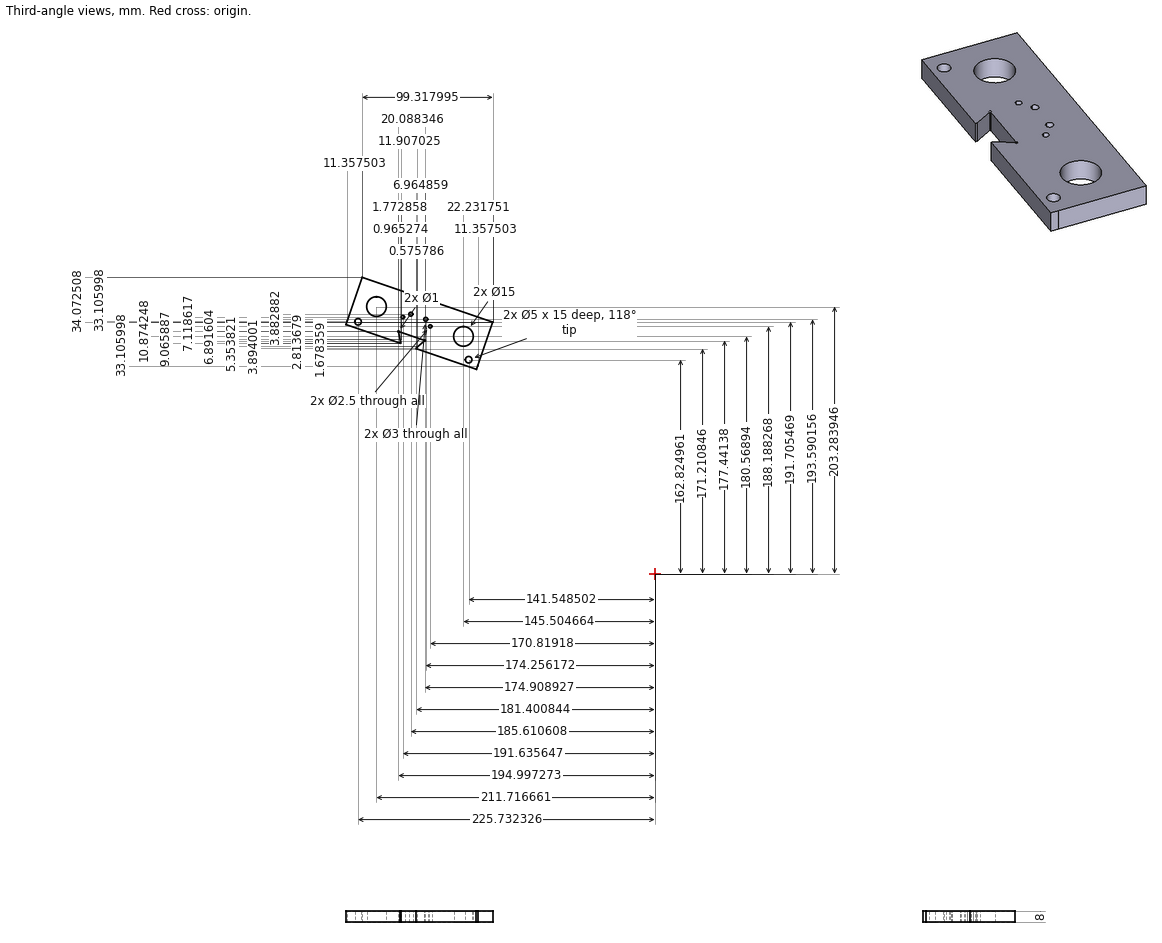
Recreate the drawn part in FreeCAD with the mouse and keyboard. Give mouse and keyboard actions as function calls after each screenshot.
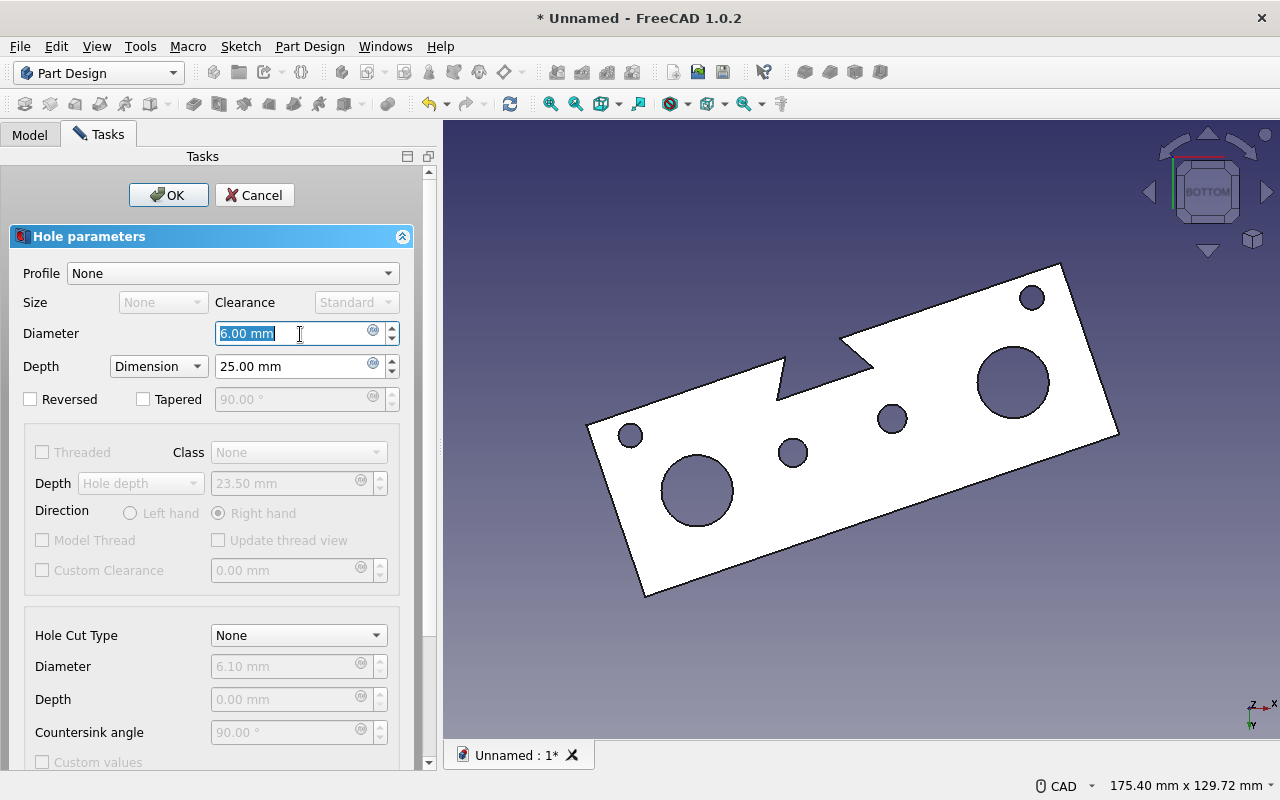
text(2.5)
key(Tab)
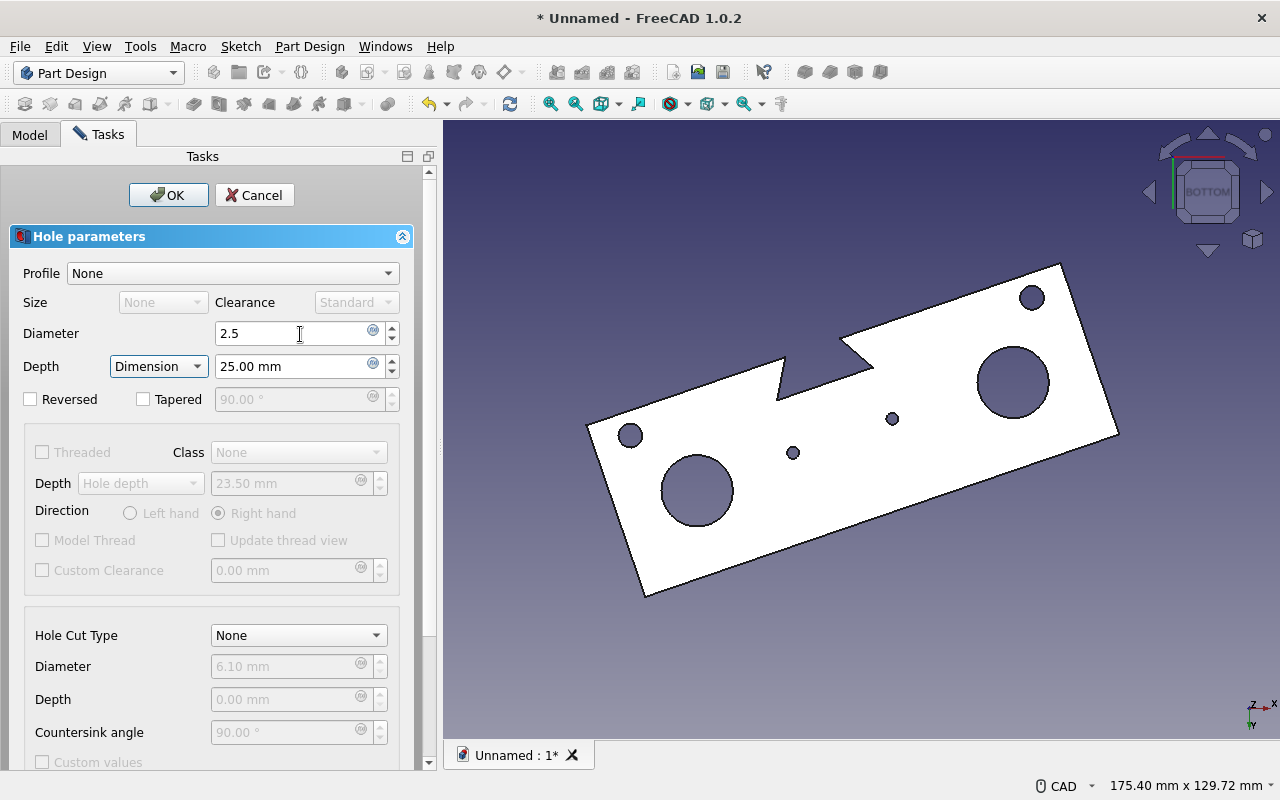
click(160, 366)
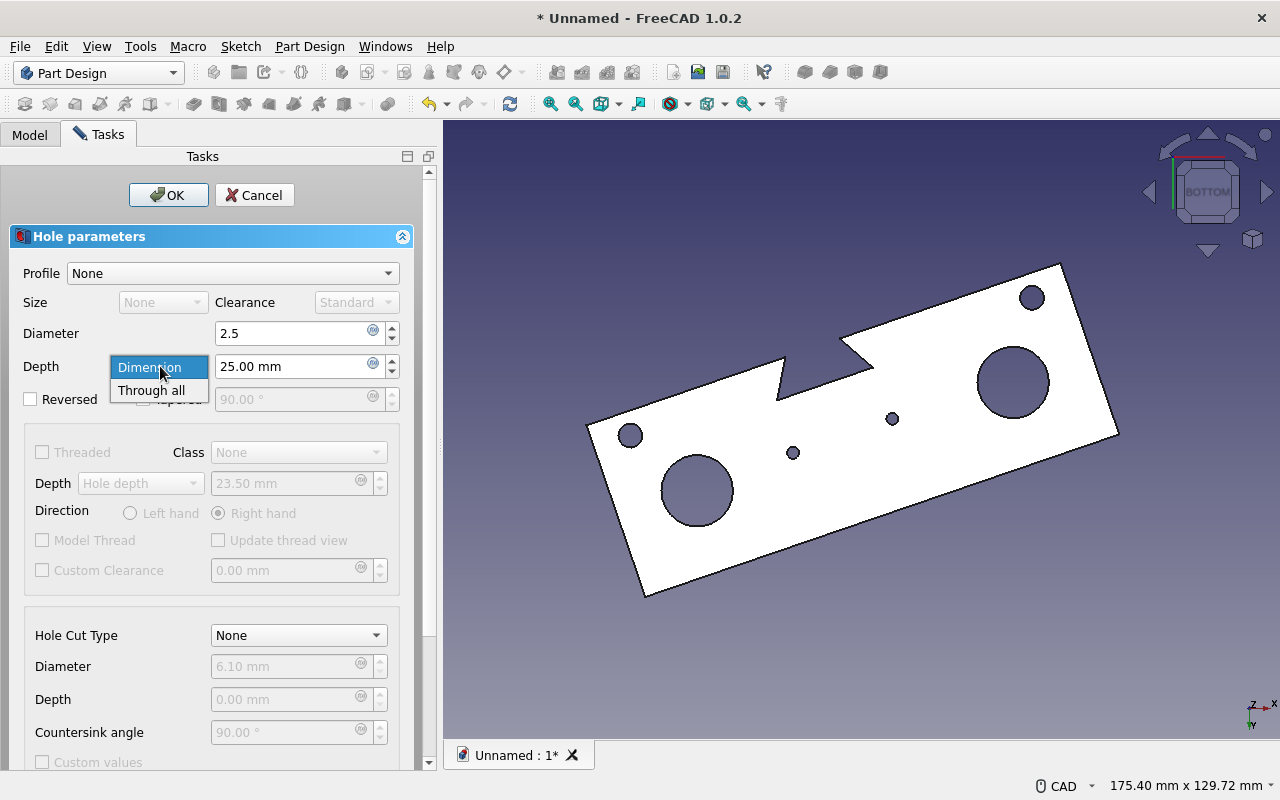
click(158, 390)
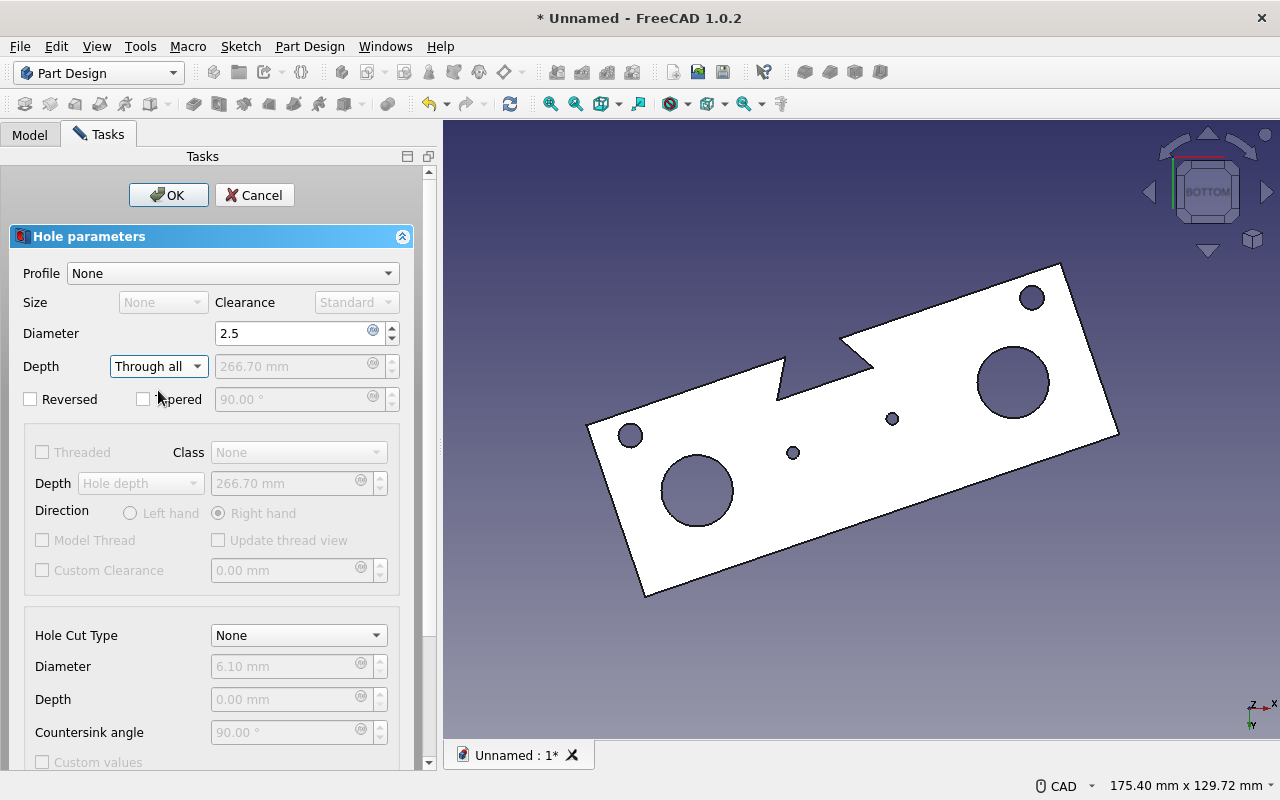
click(169, 195)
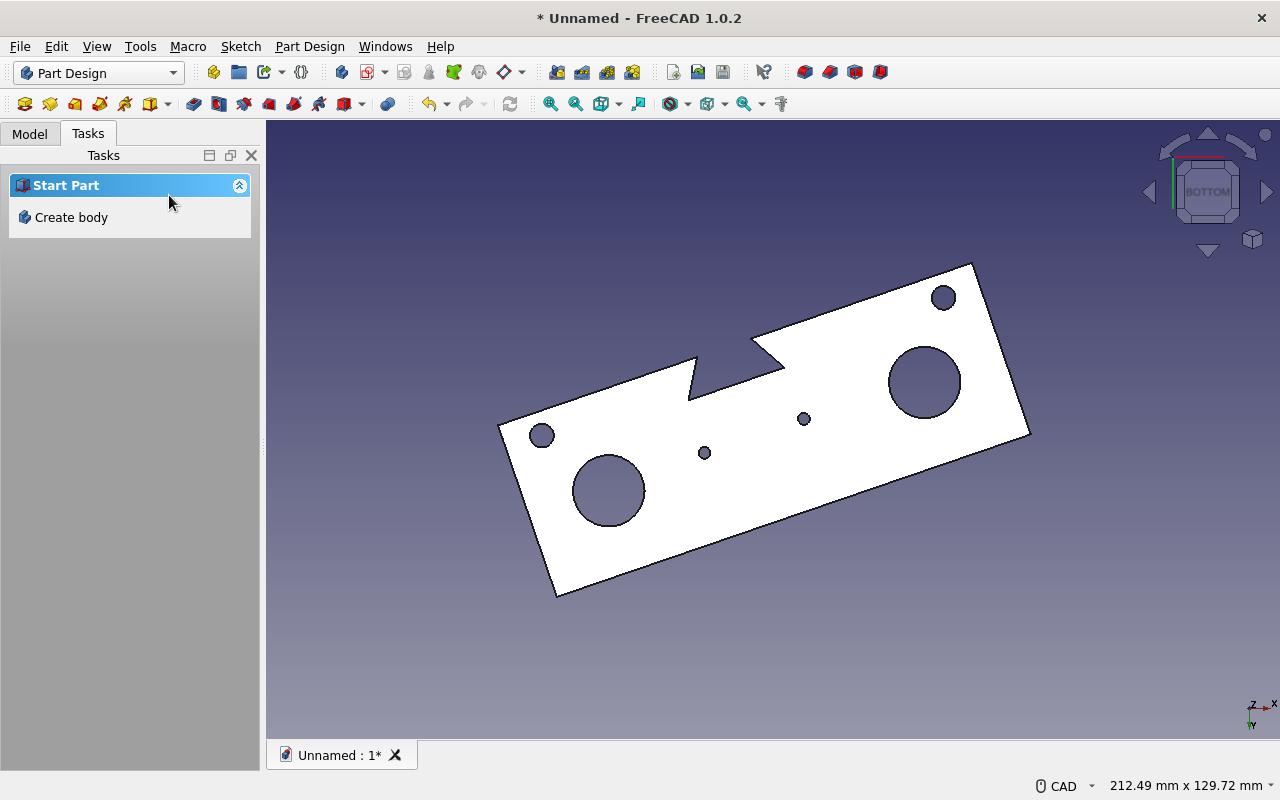
click(840, 381)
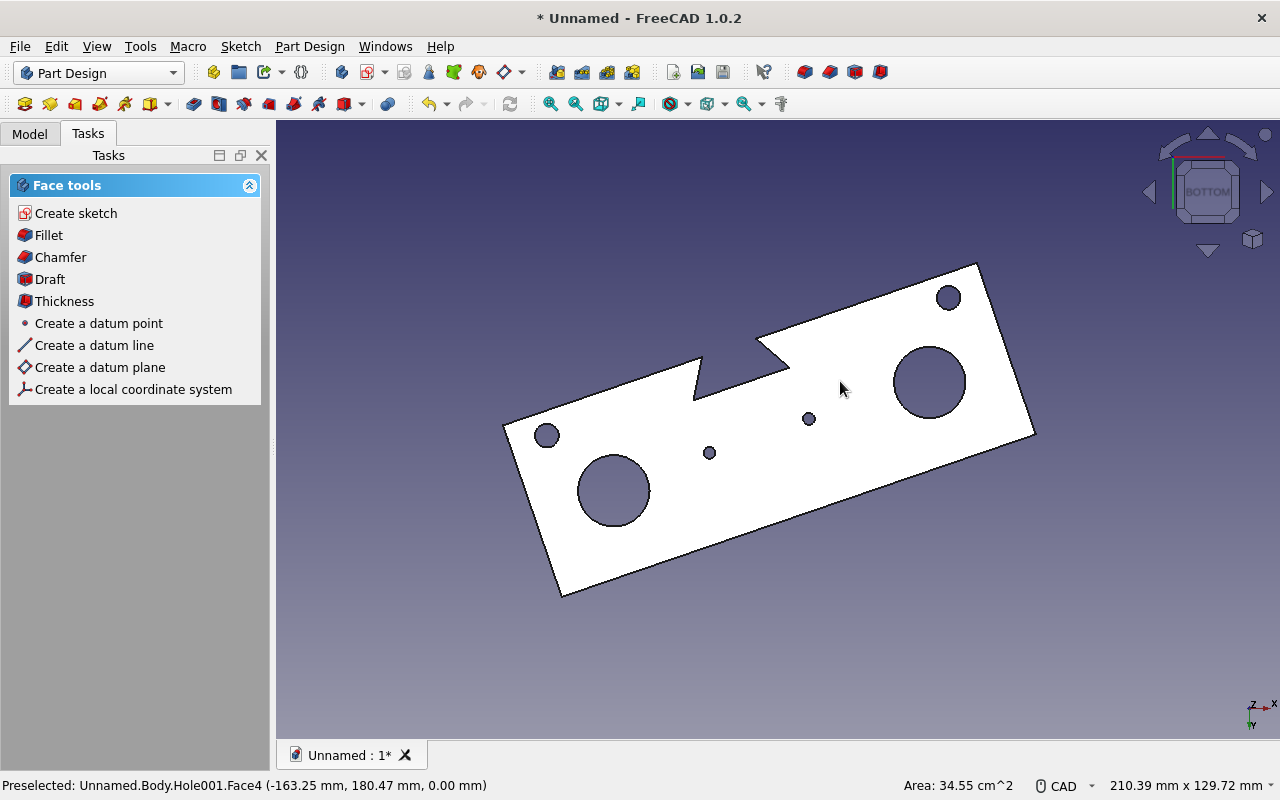
click(366, 72)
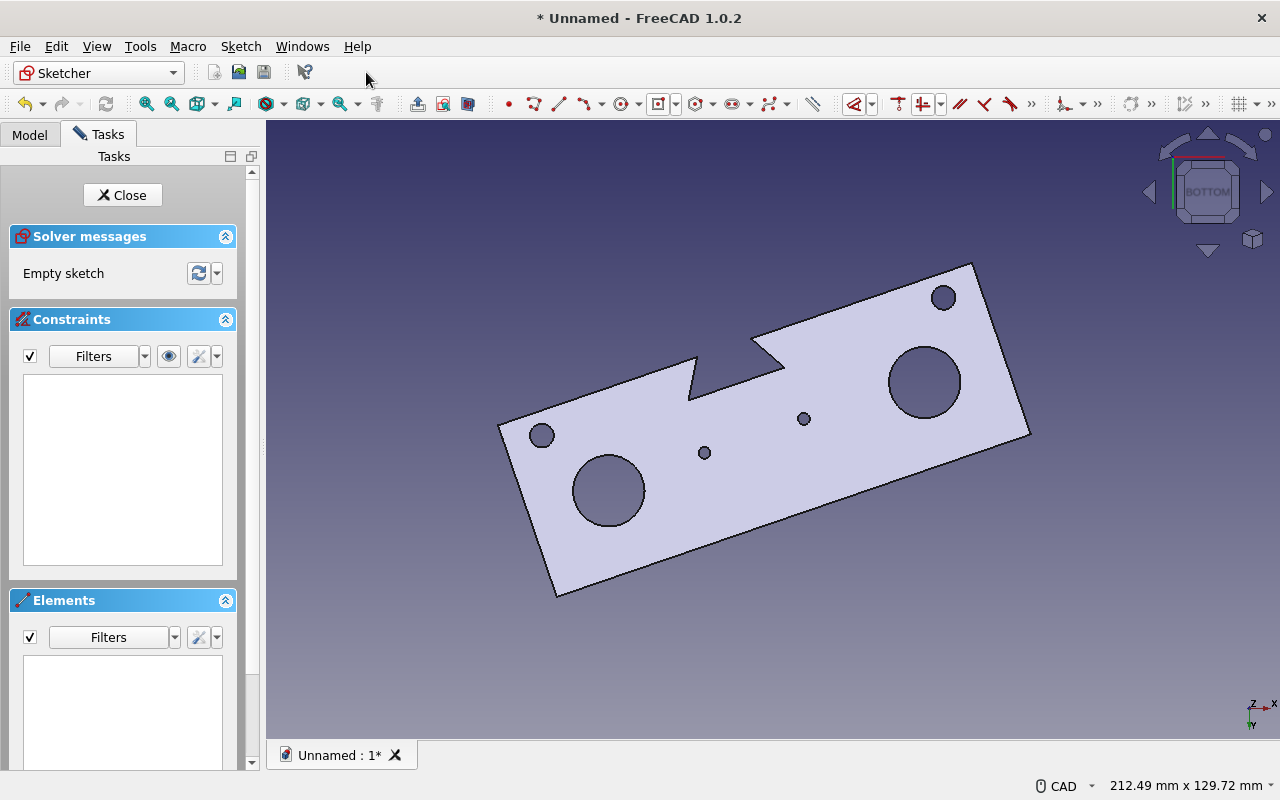
scroll(767, 457, up, 11)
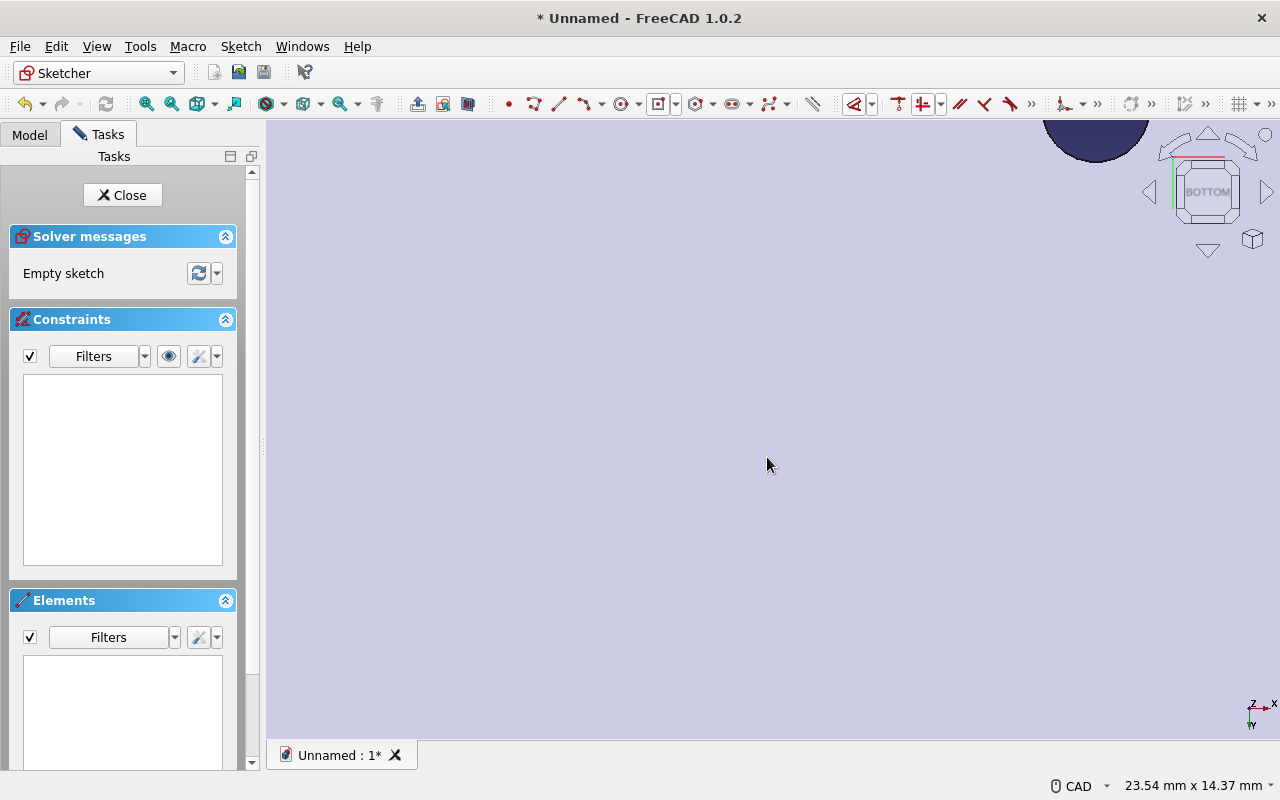
click(620, 104)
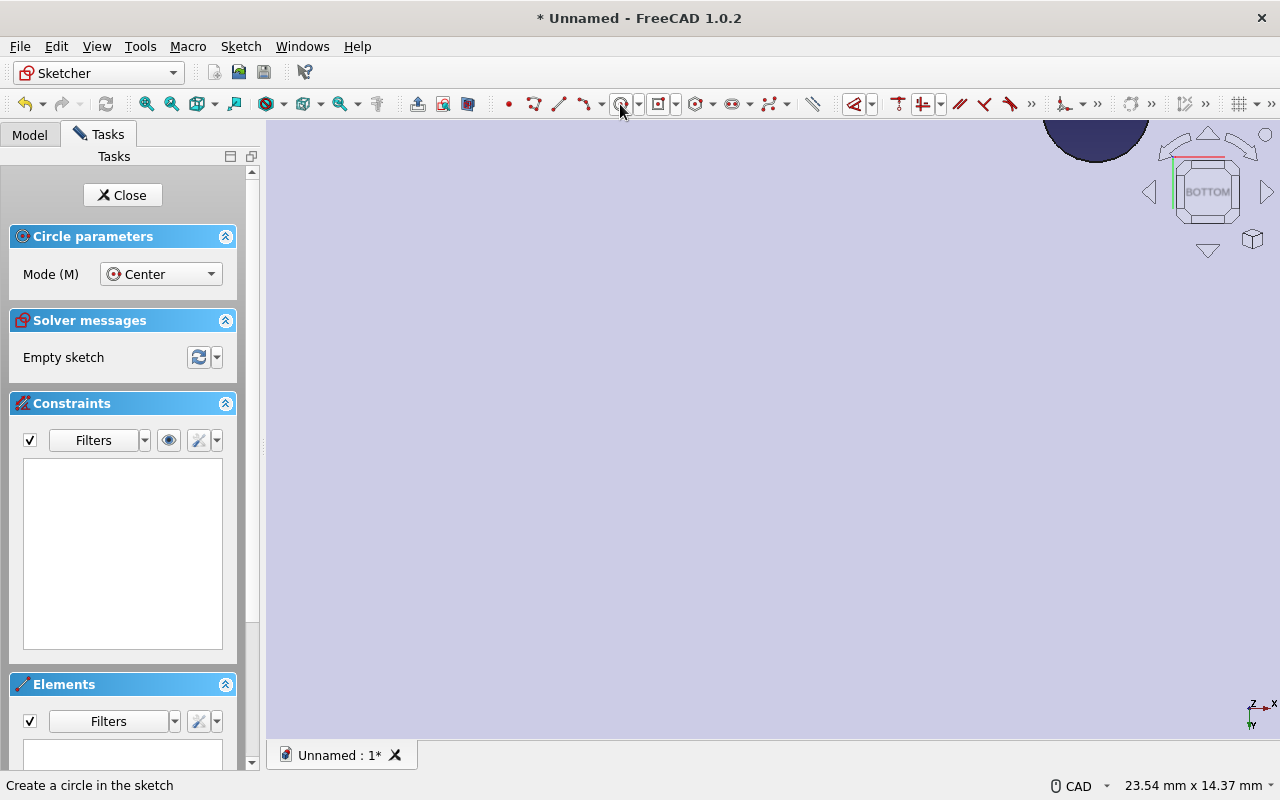
click(948, 341)
click(994, 295)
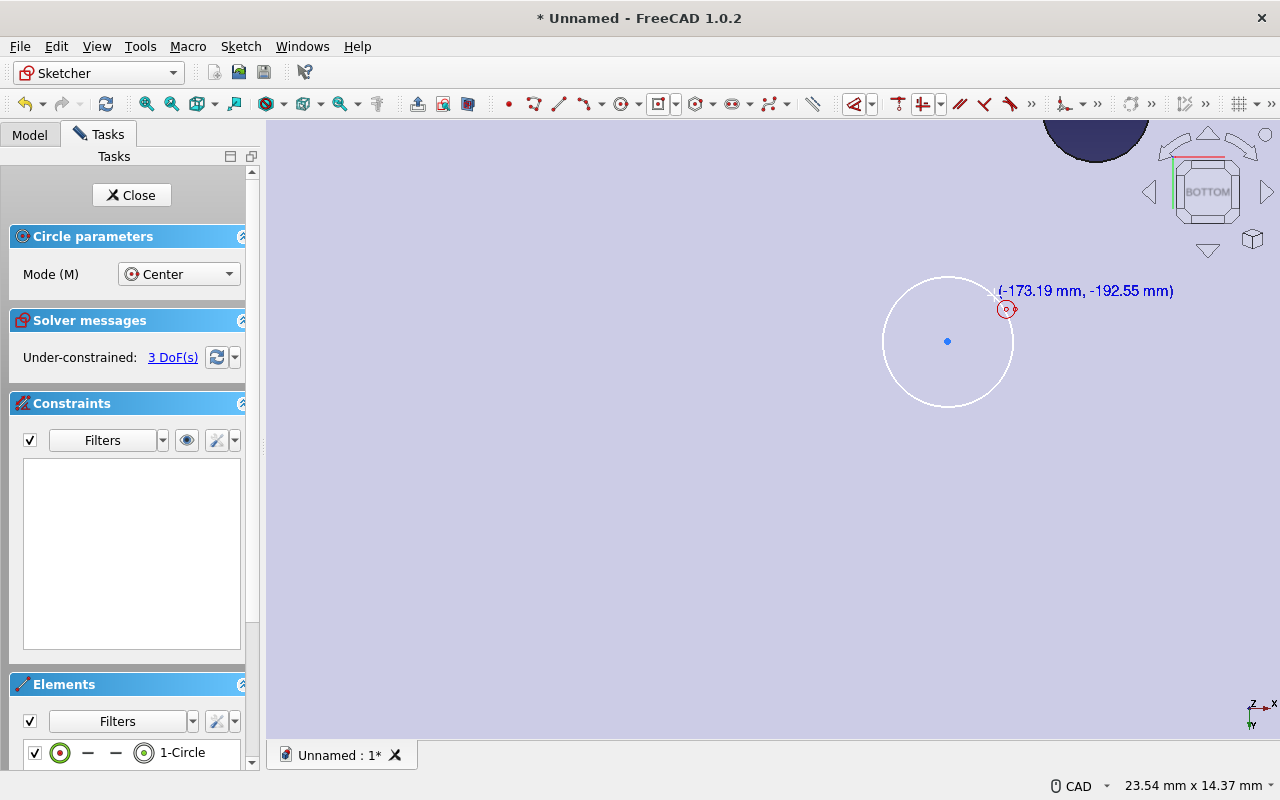
click(459, 508)
click(505, 462)
key(Escape)